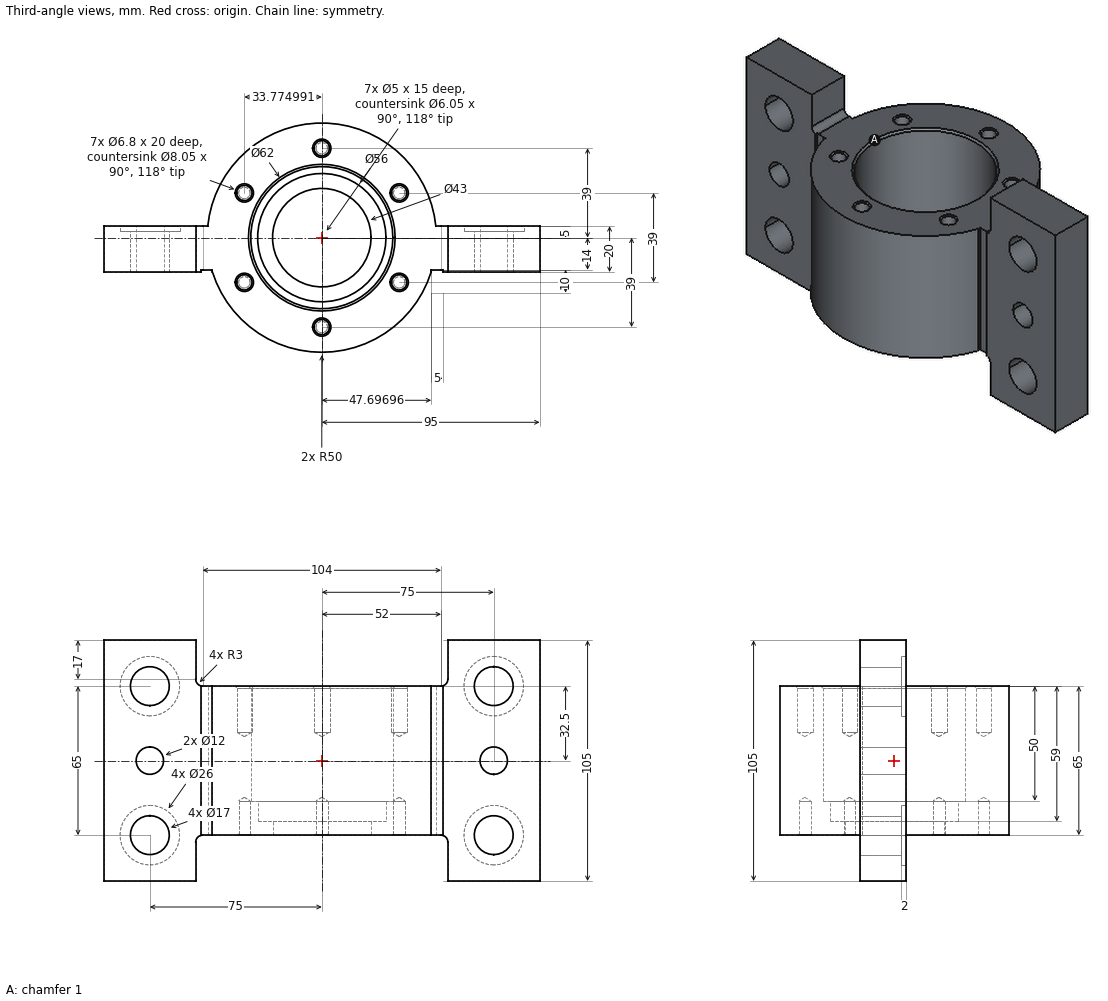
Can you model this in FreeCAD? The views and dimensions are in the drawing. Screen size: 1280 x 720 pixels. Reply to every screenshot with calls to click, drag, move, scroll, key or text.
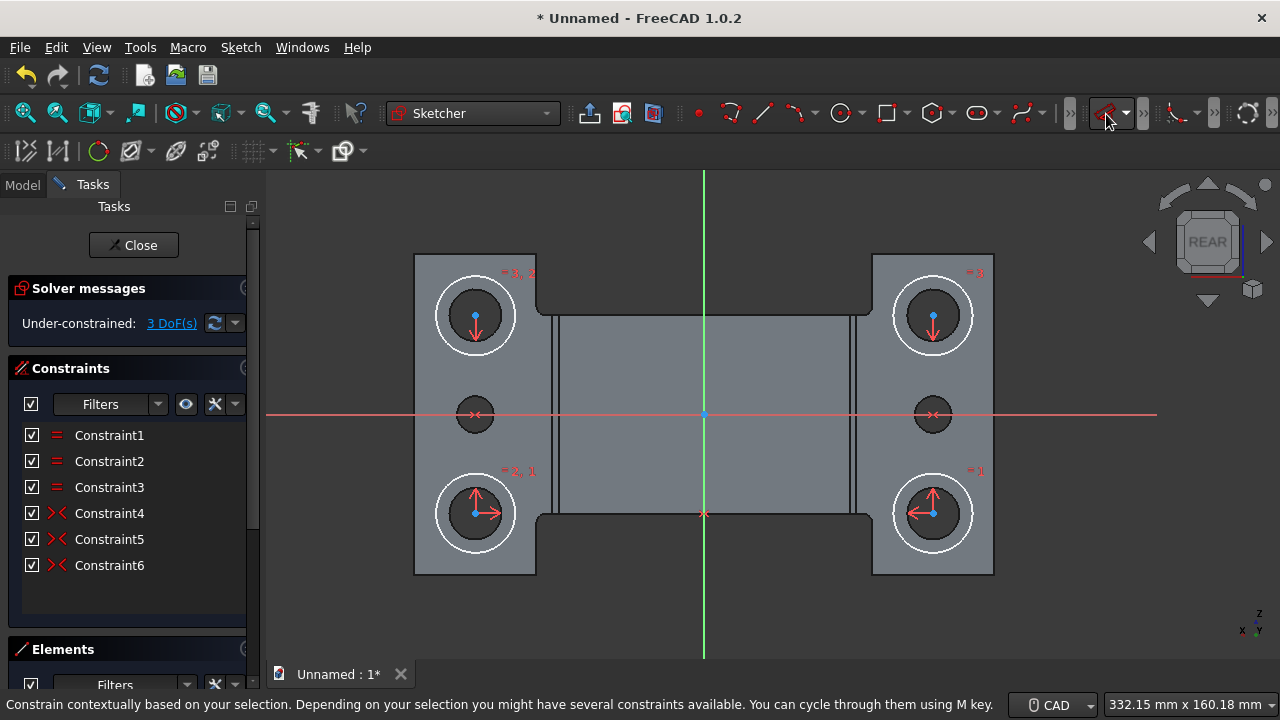
click(961, 485)
click(984, 462)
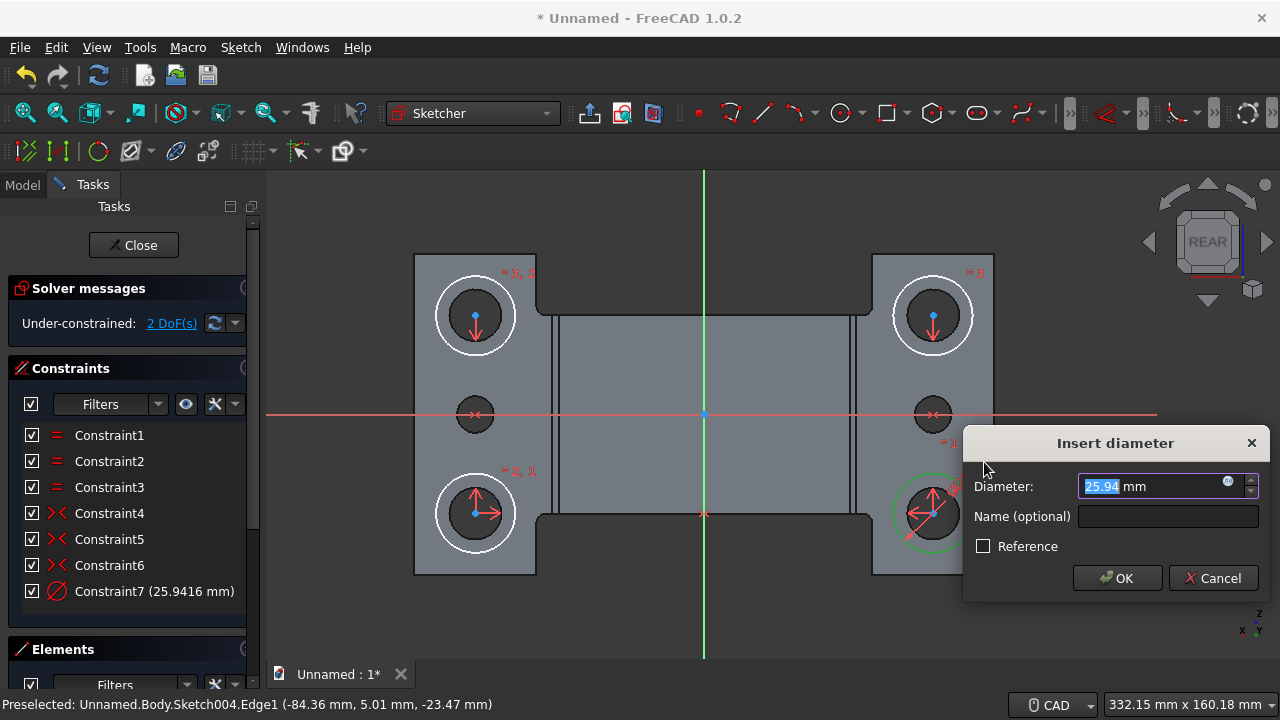
text(26)
key(Return)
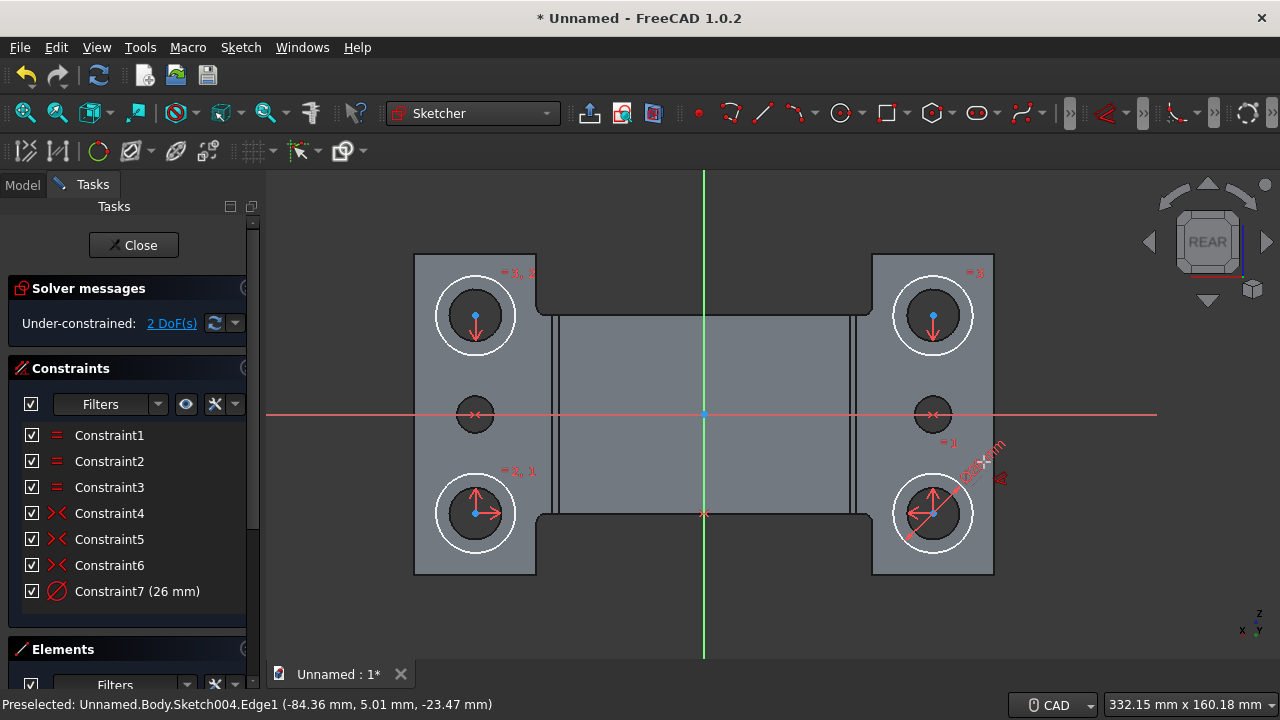
click(933, 513)
click(819, 547)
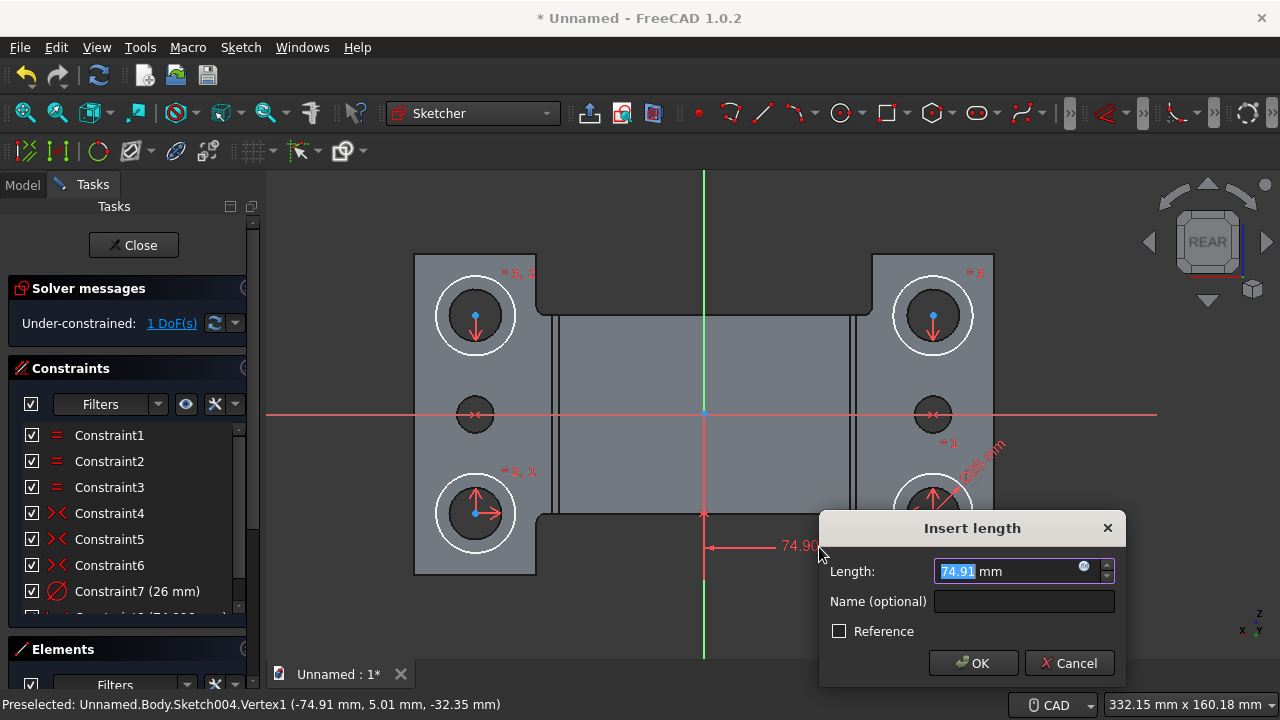
text(75)
key(Return)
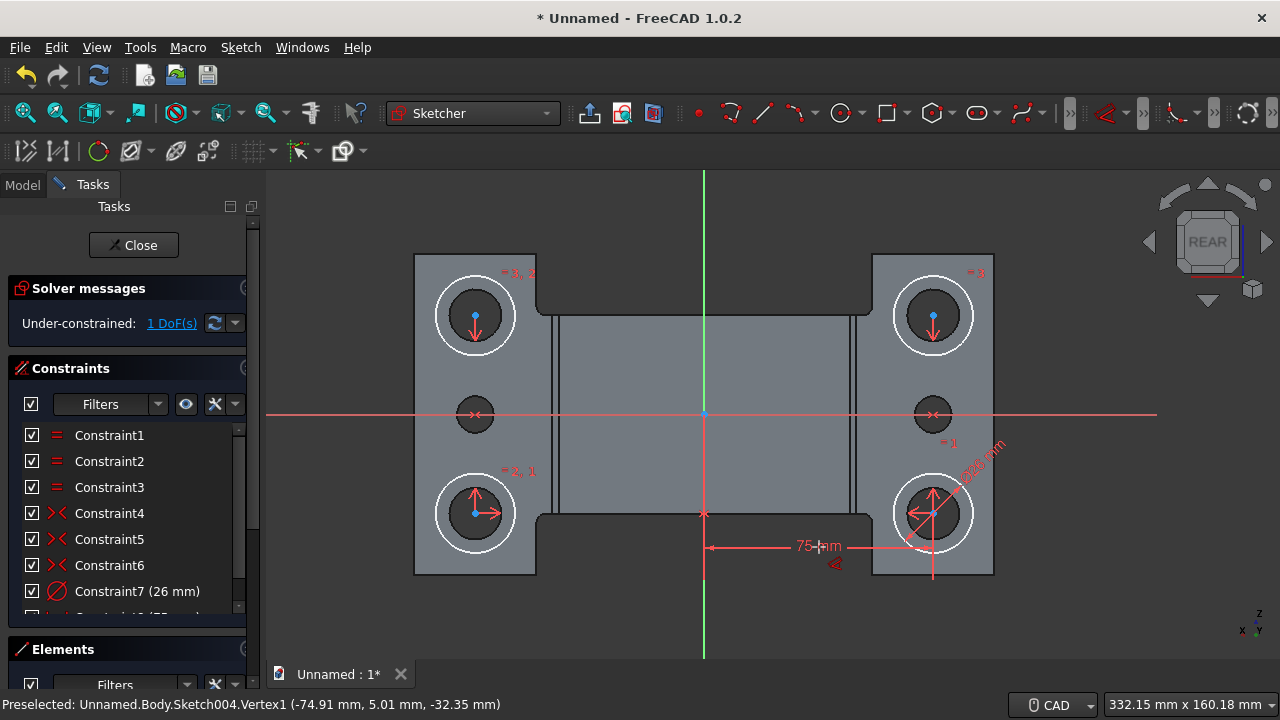
click(475, 513)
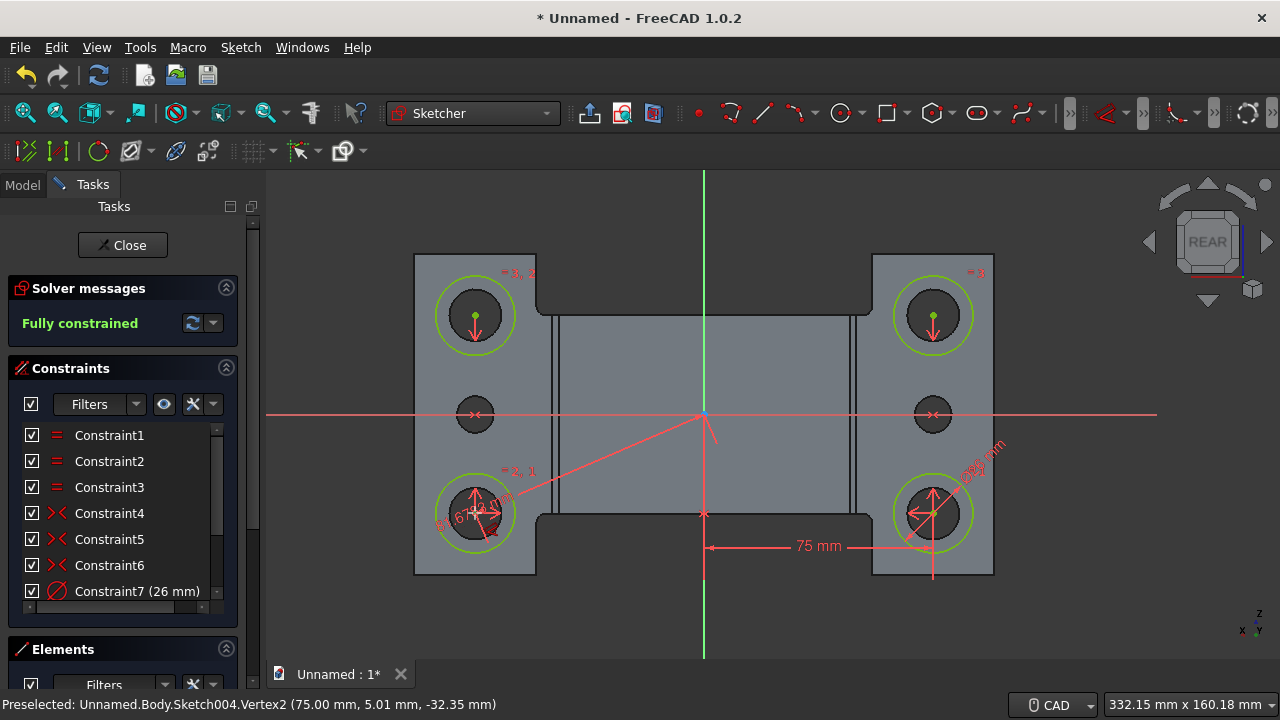
click(475, 316)
click(441, 369)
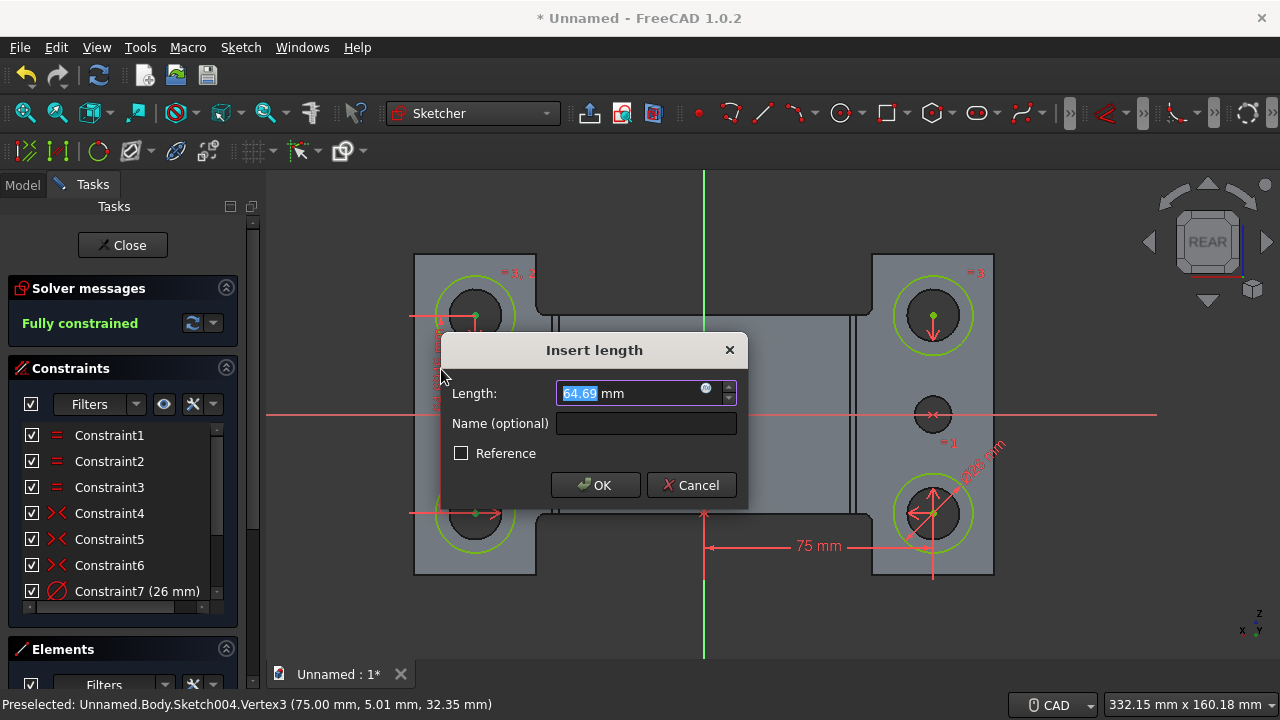
text(65)
key(Return)
key(Escape)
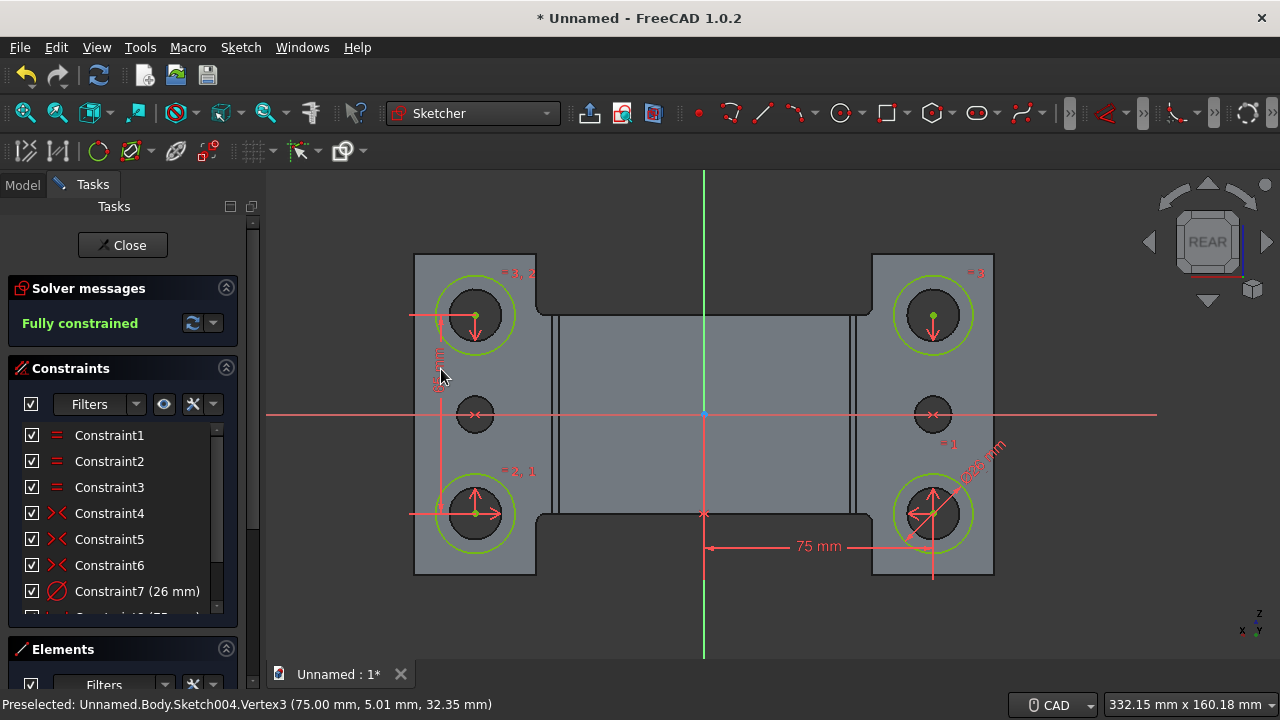
click(123, 245)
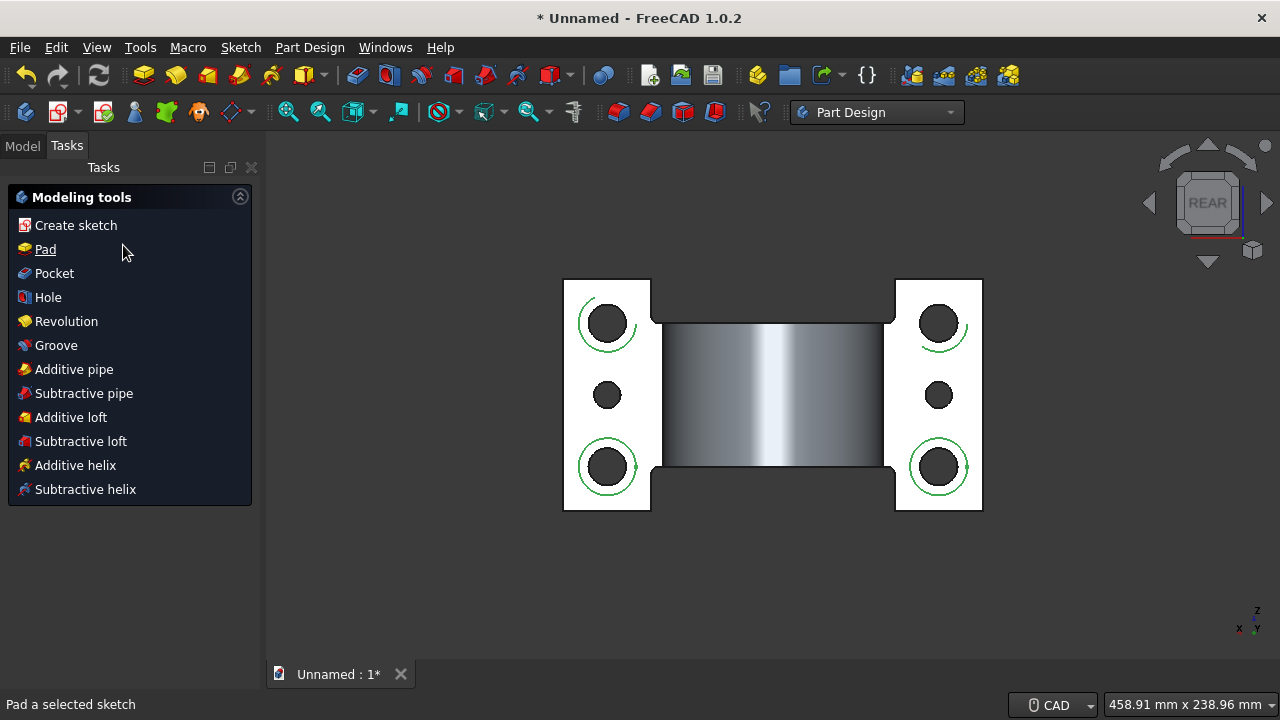
click(358, 76)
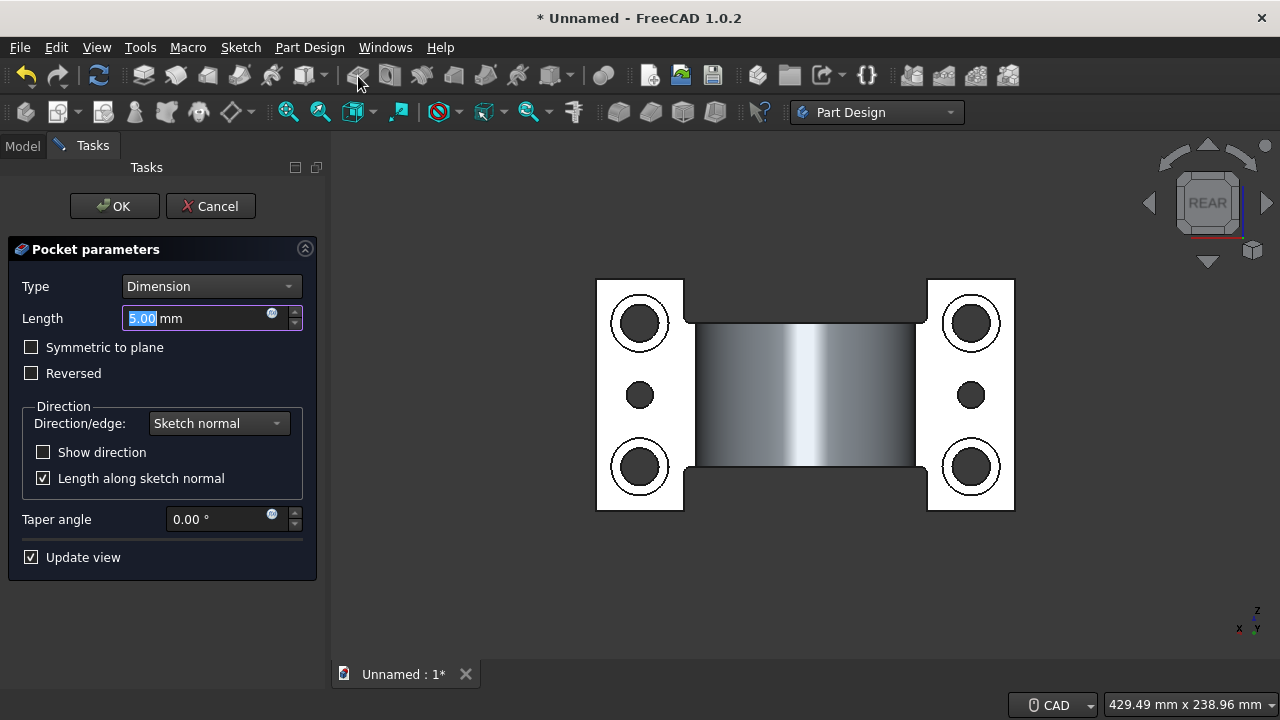
text(2)
key(Tab)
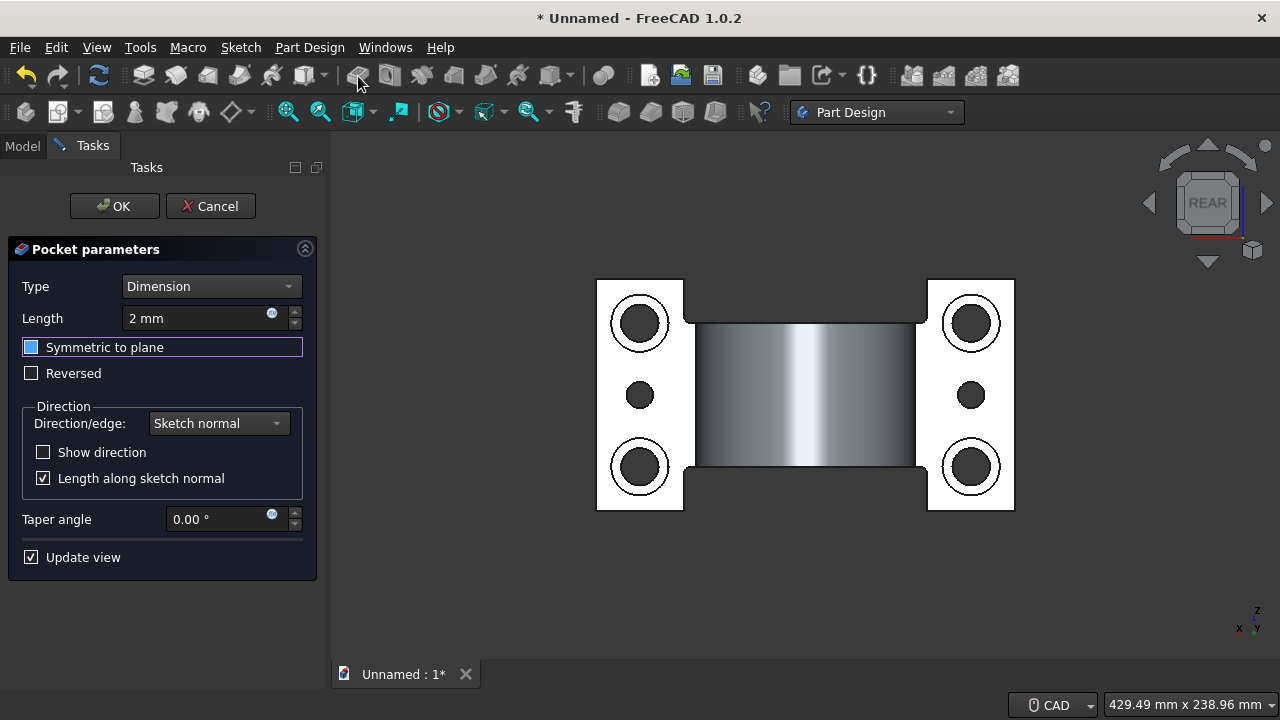
click(115, 206)